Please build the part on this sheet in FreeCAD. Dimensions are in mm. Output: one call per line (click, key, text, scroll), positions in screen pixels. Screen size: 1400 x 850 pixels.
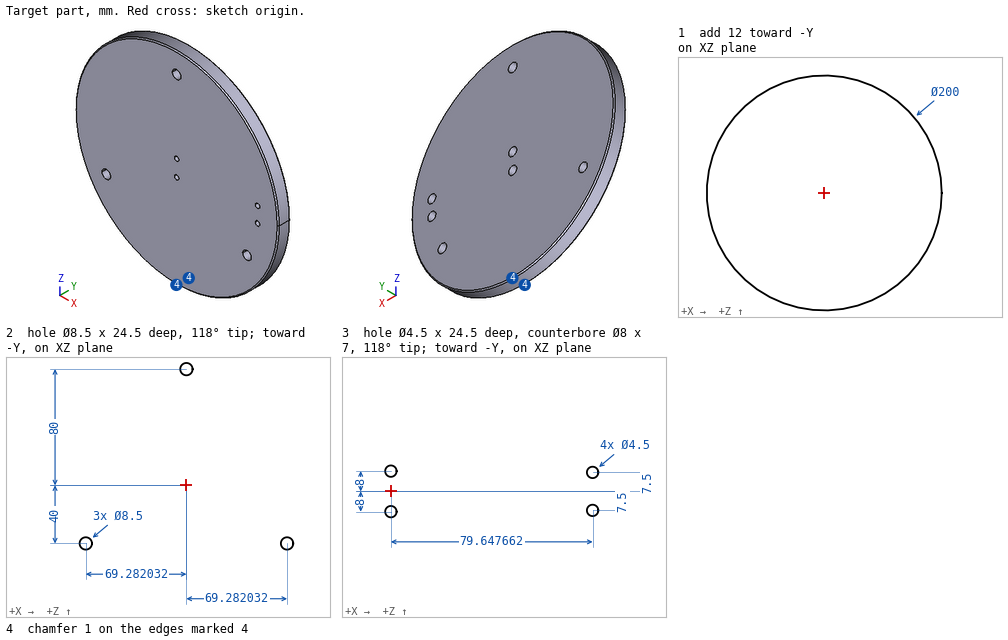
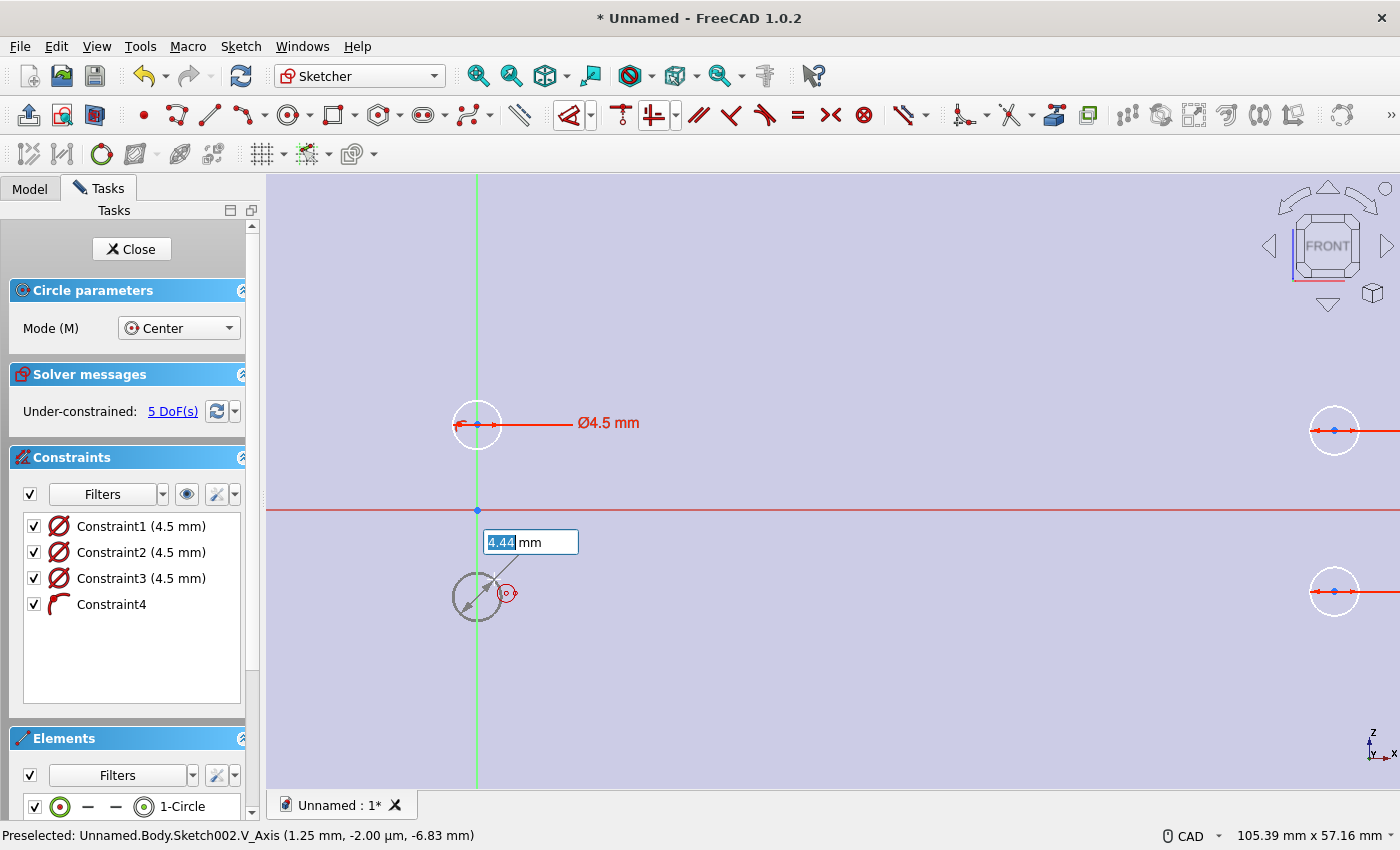
text(4.5)
key(Return)
key(Escape)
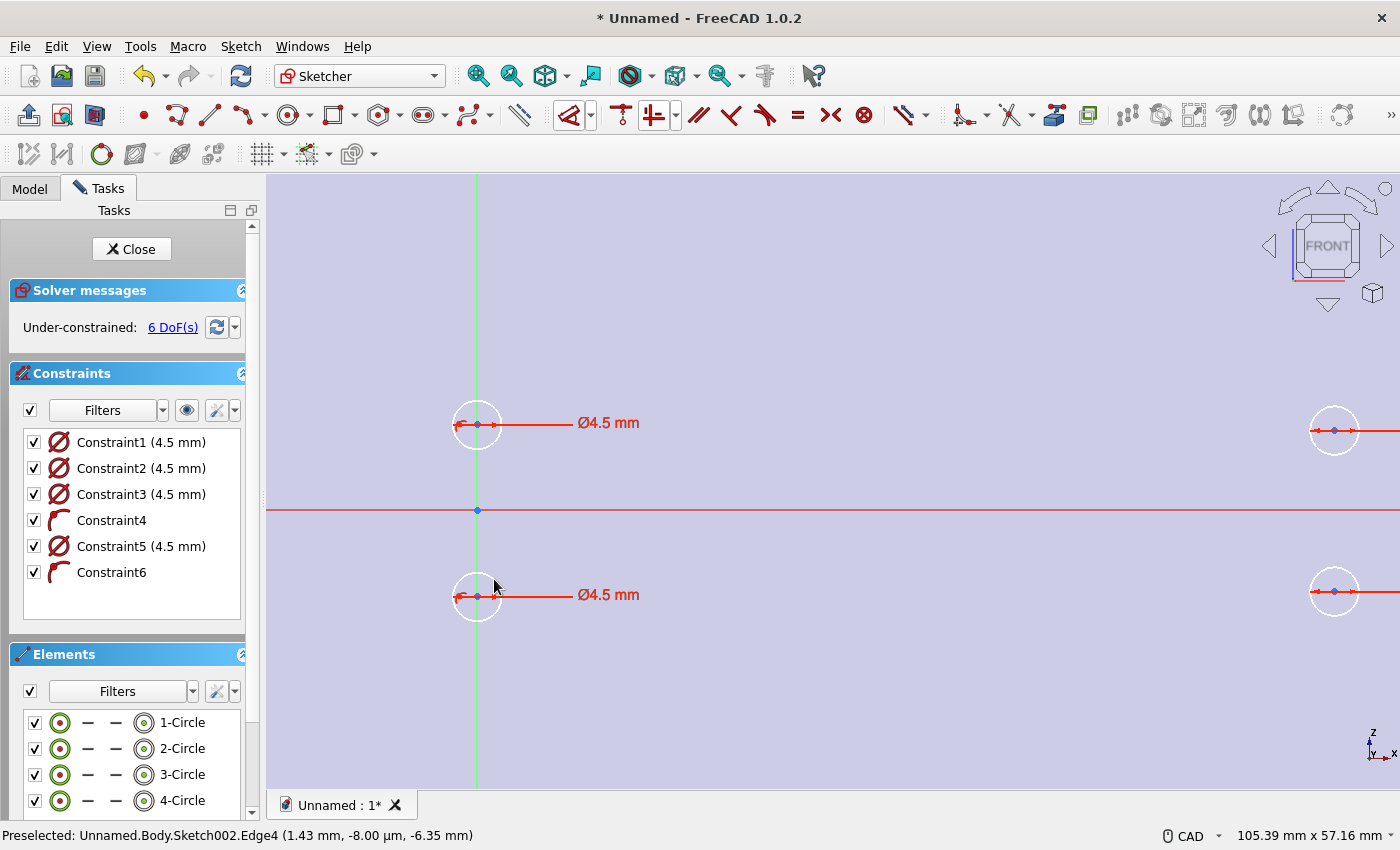
scroll(477, 423, down, 2)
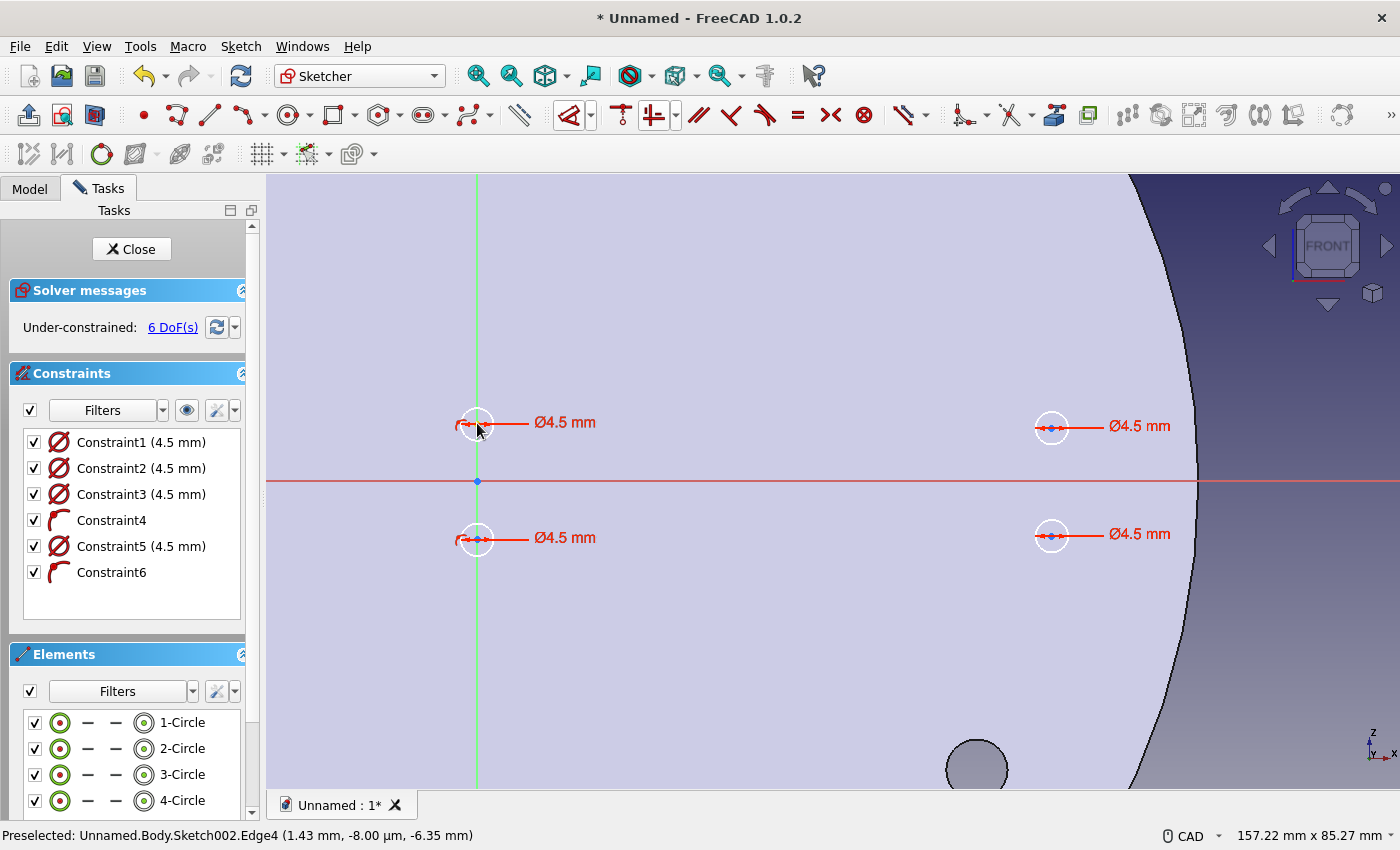
click(1052, 536)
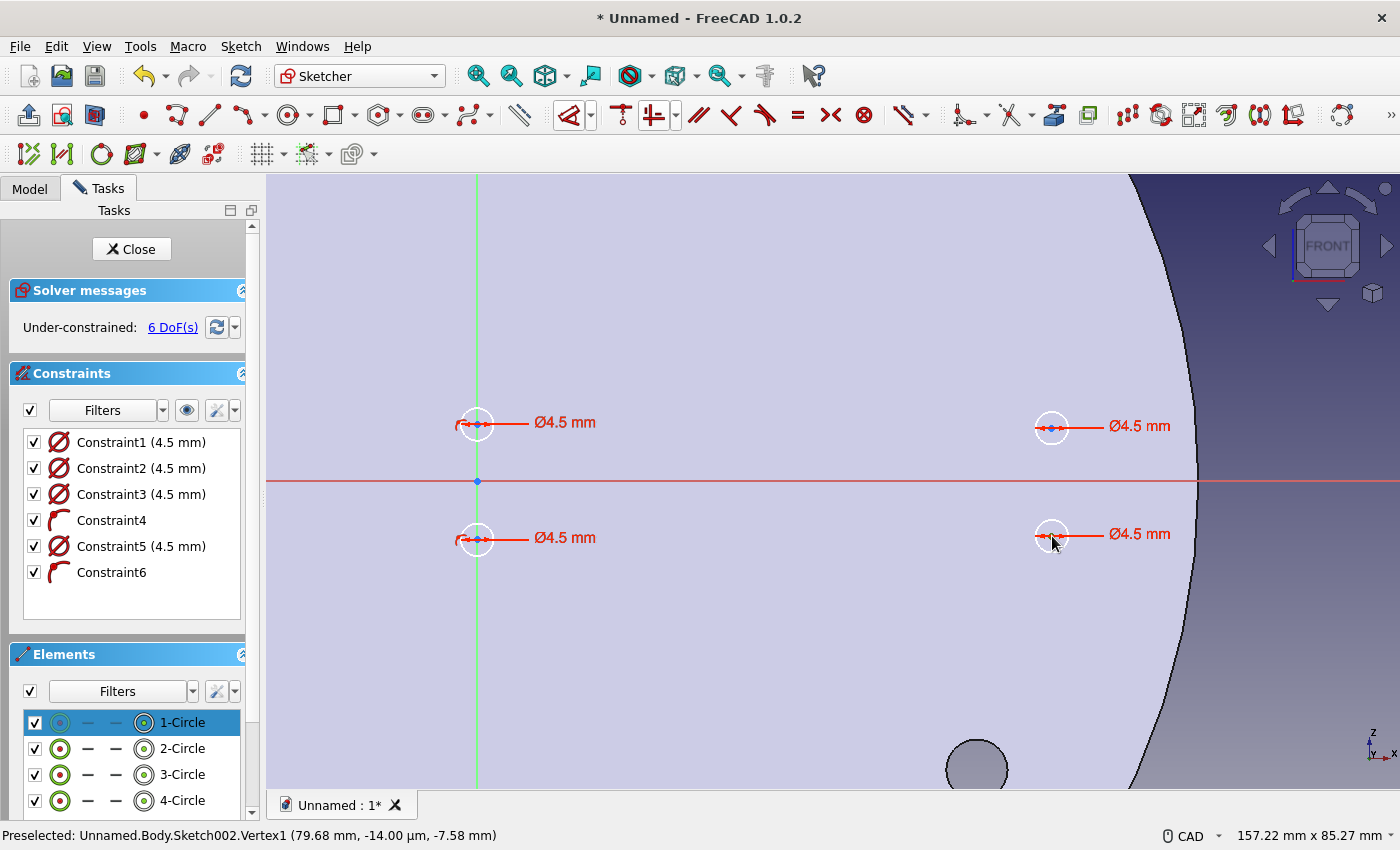
click(1052, 428)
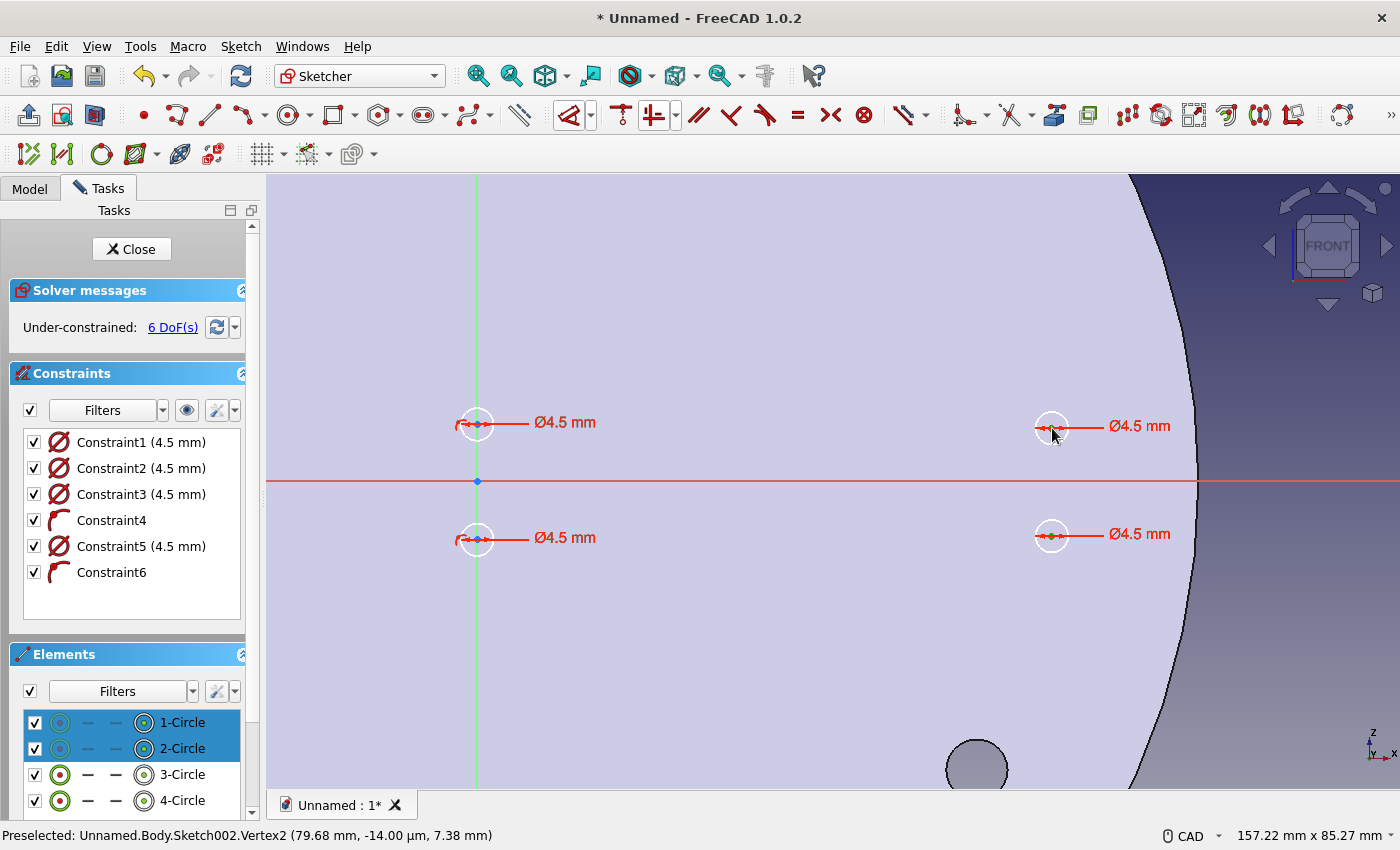
key(v)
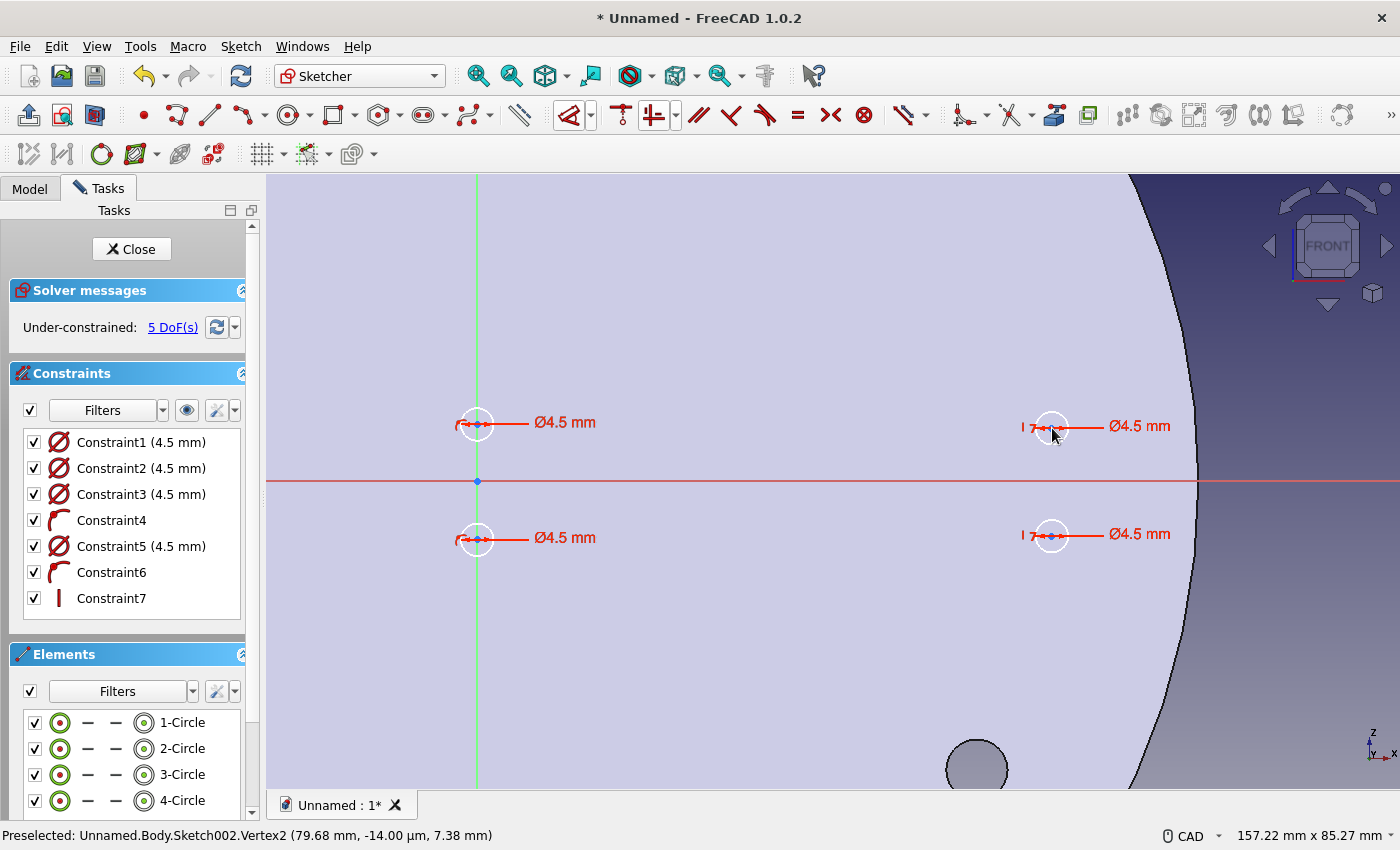
click(477, 424)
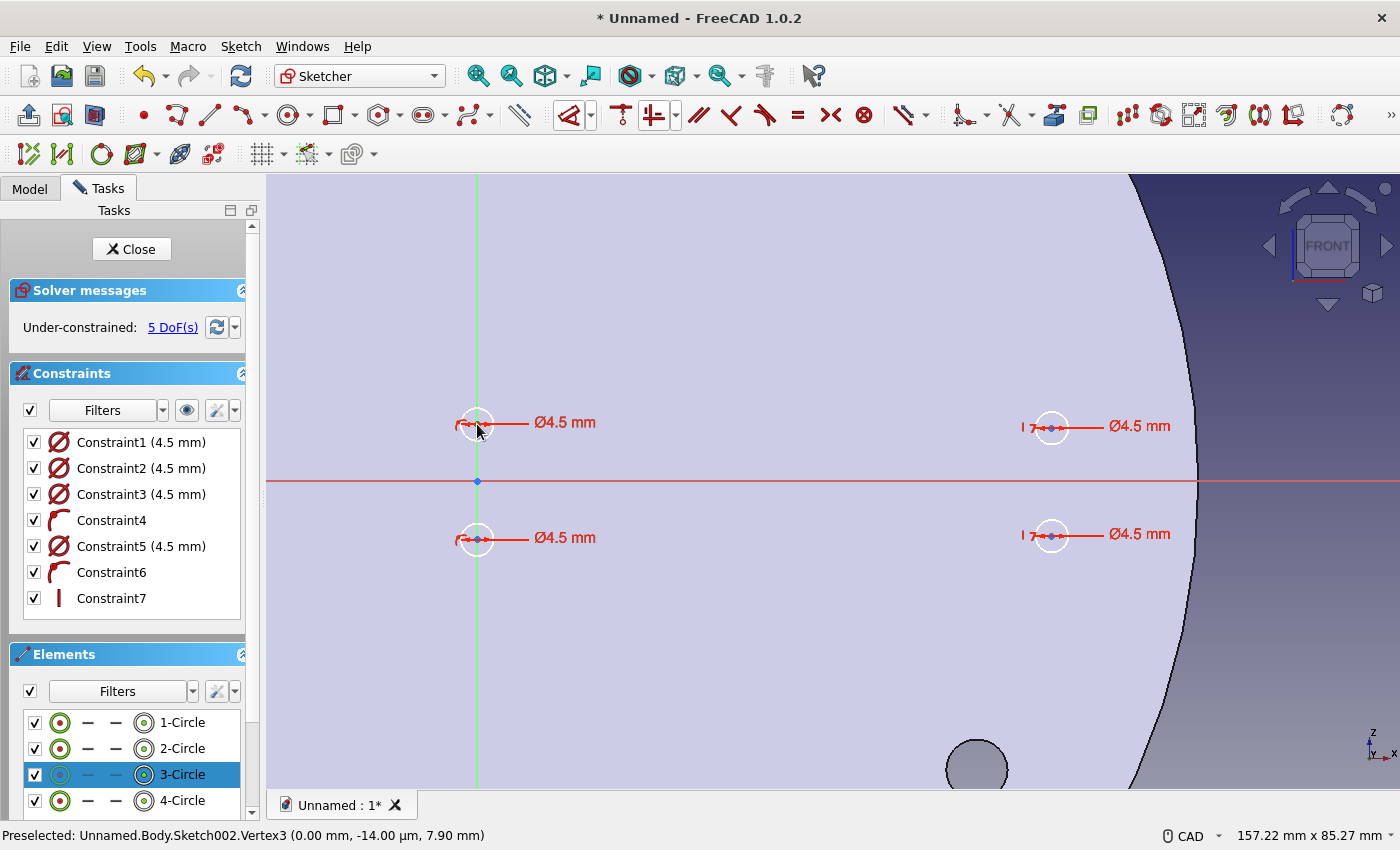
key(i)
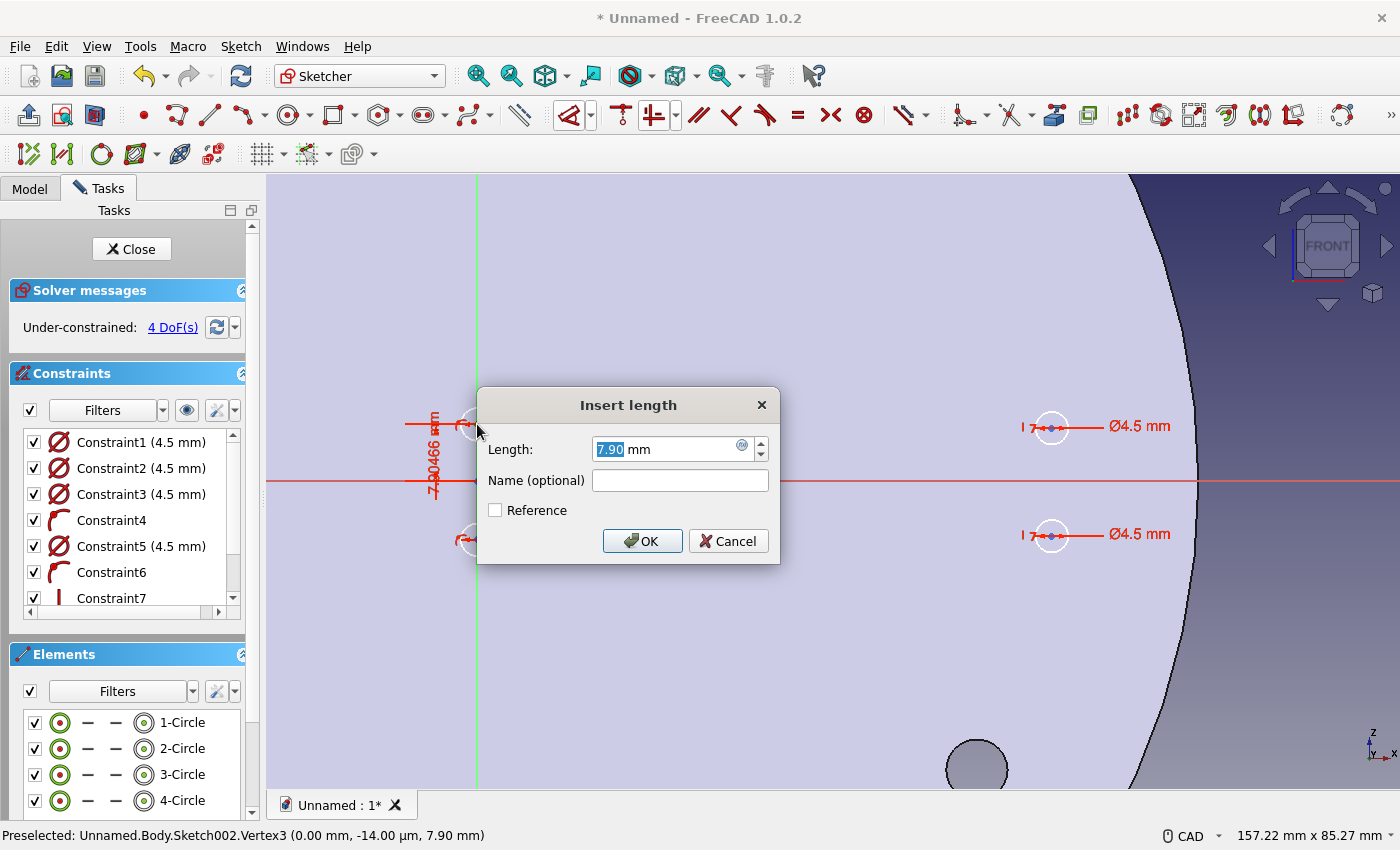
text(8)
key(Return)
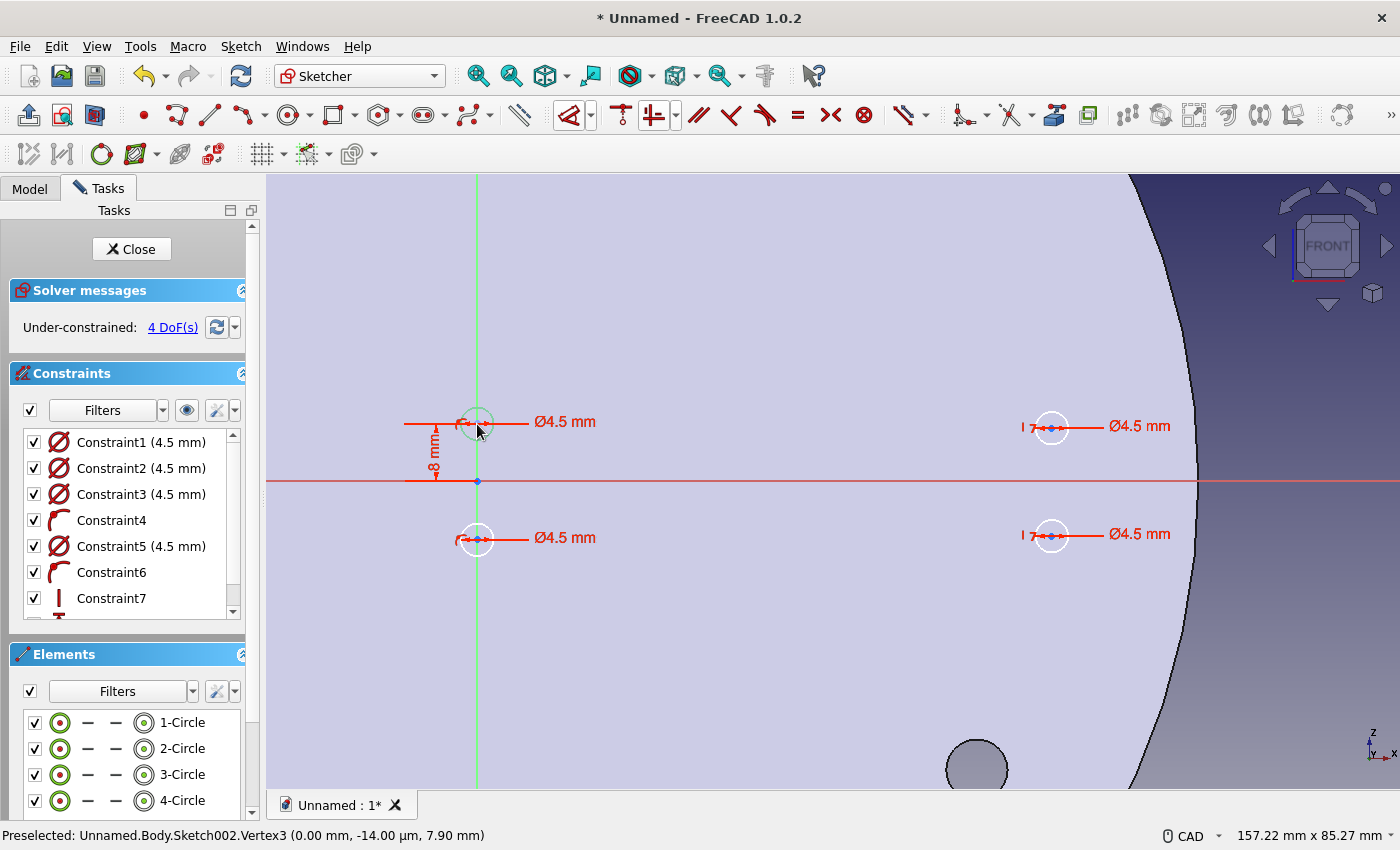
click(477, 540)